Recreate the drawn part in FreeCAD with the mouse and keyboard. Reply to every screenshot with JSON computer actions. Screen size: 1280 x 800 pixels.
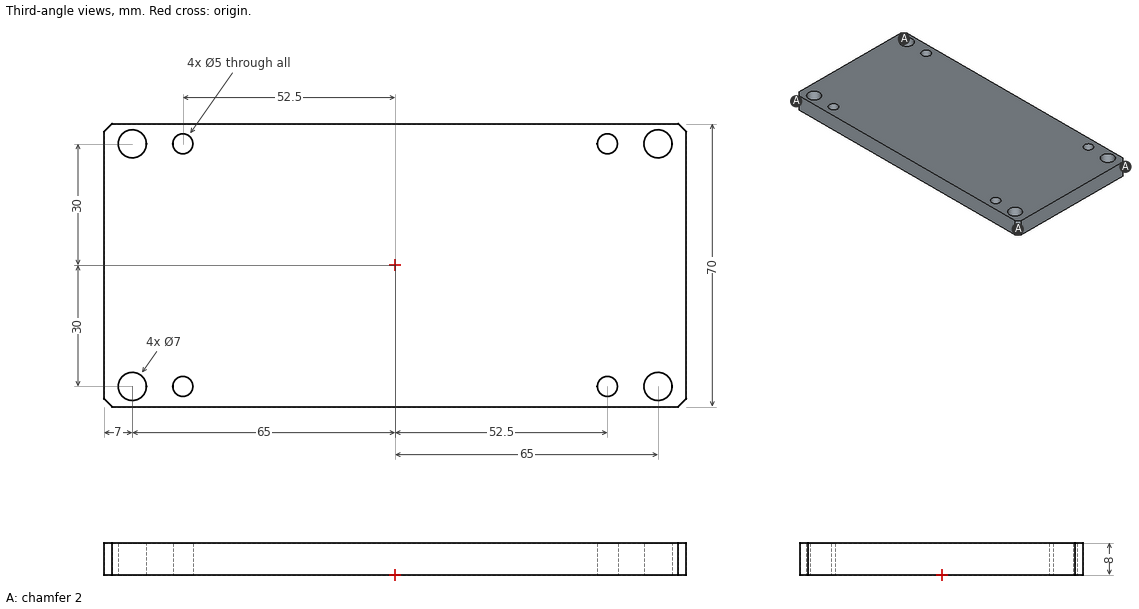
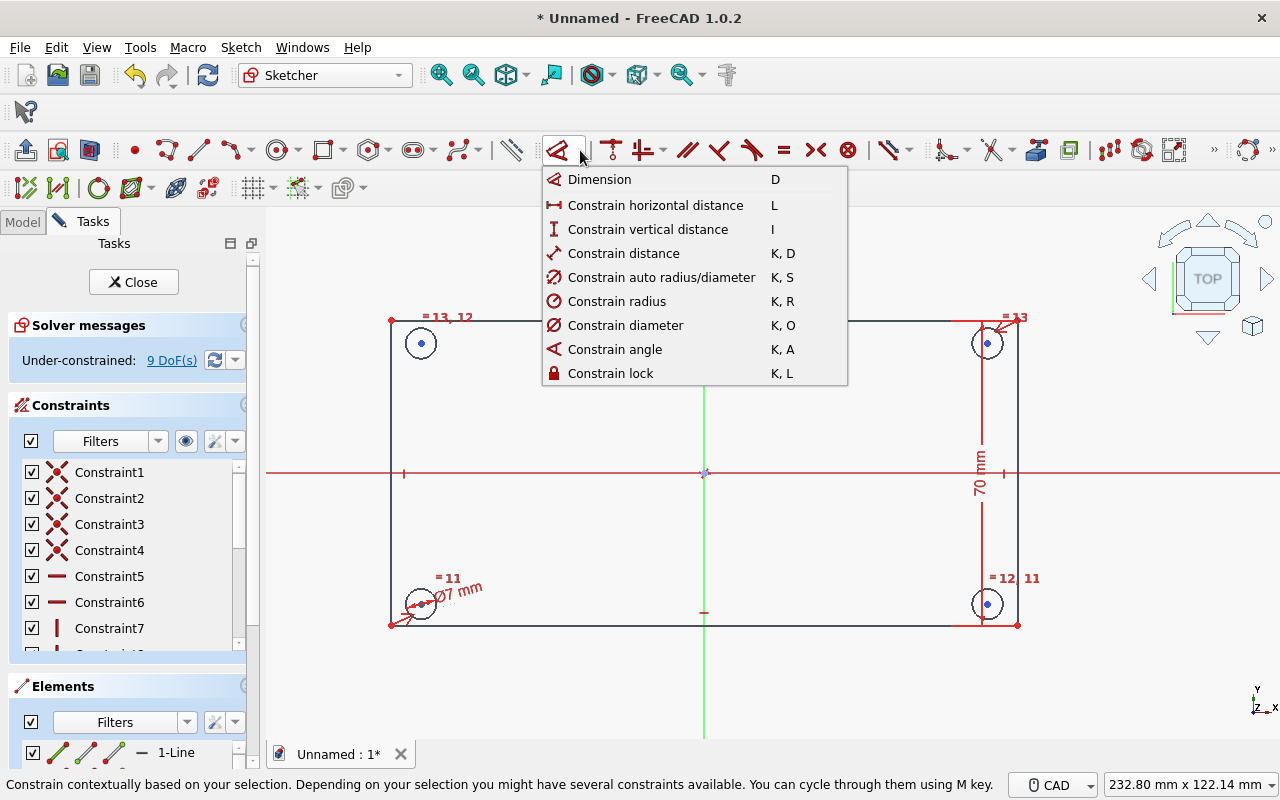
{"action": "left_click", "coordinate": [695, 205]}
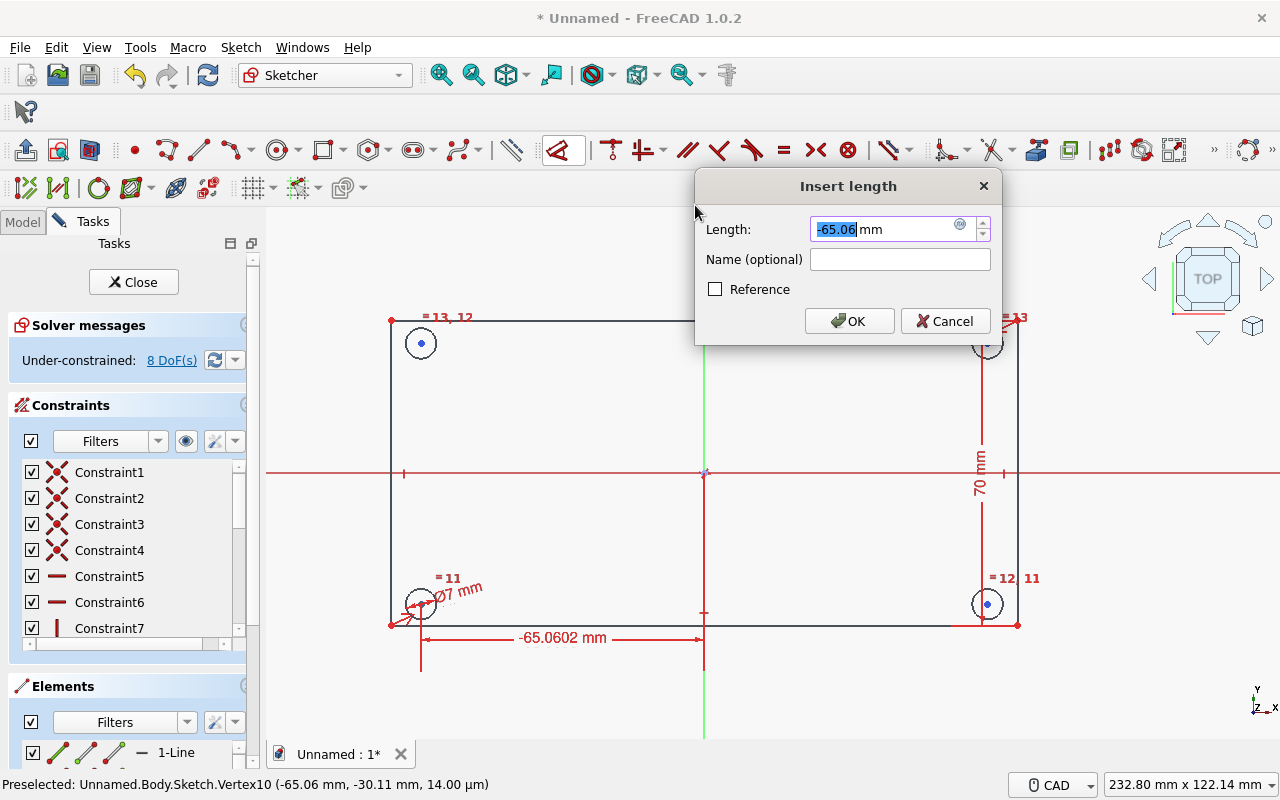
{"action": "type", "text": "-65"}
{"action": "key", "text": "Return"}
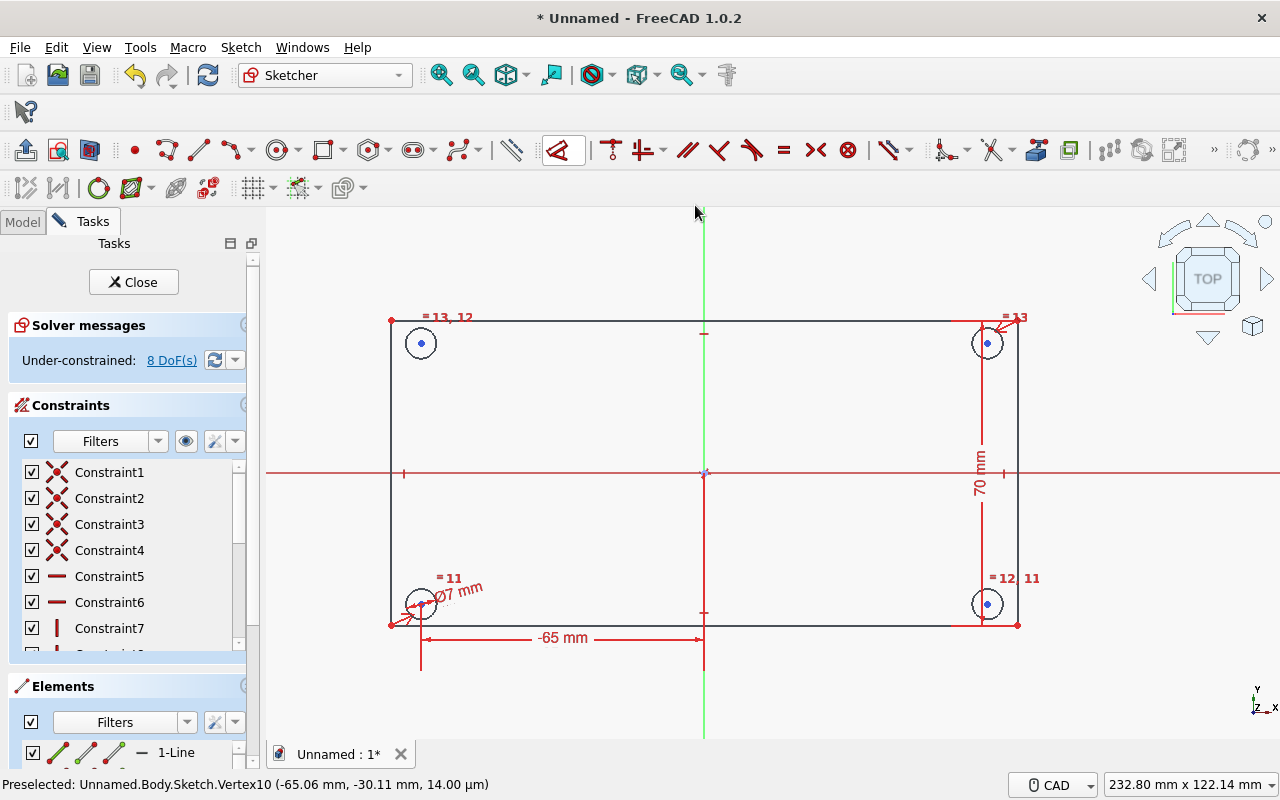
{"action": "left_click", "coordinate": [421, 604]}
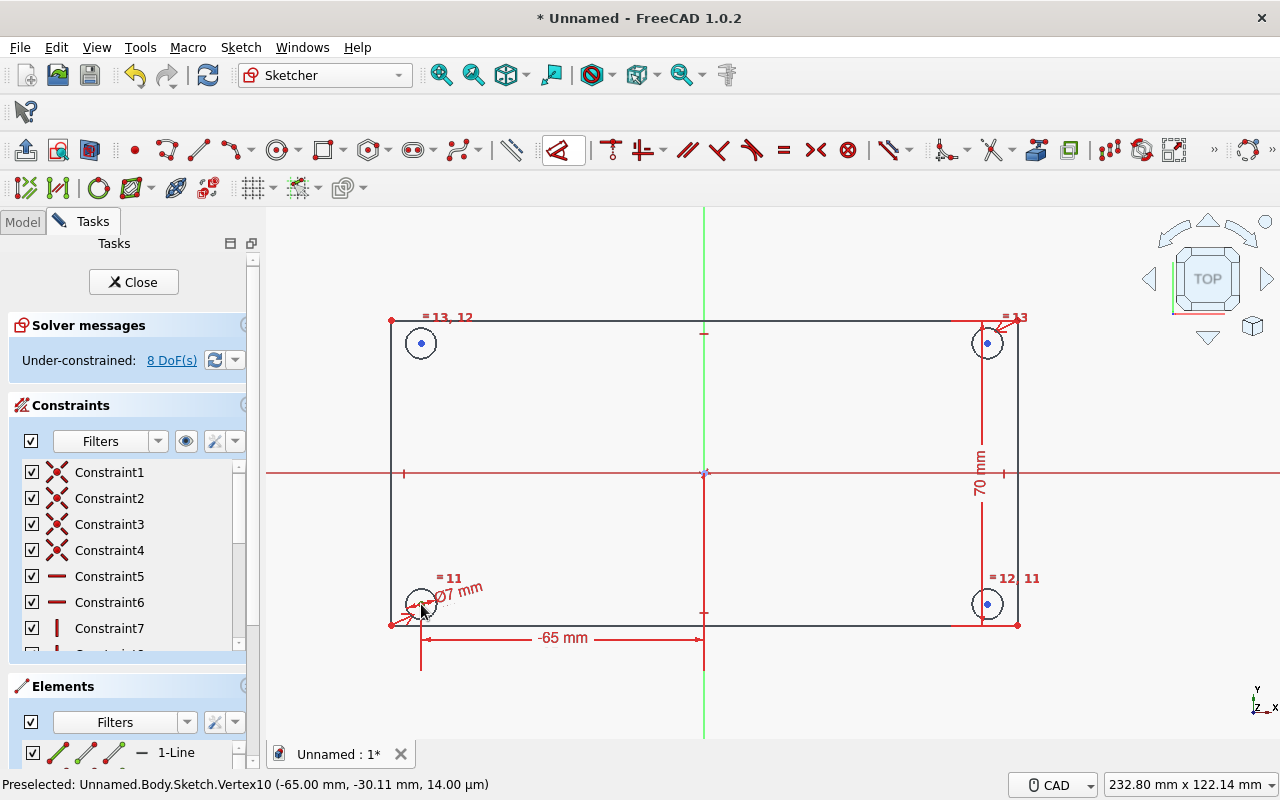
{"action": "key", "text": "i"}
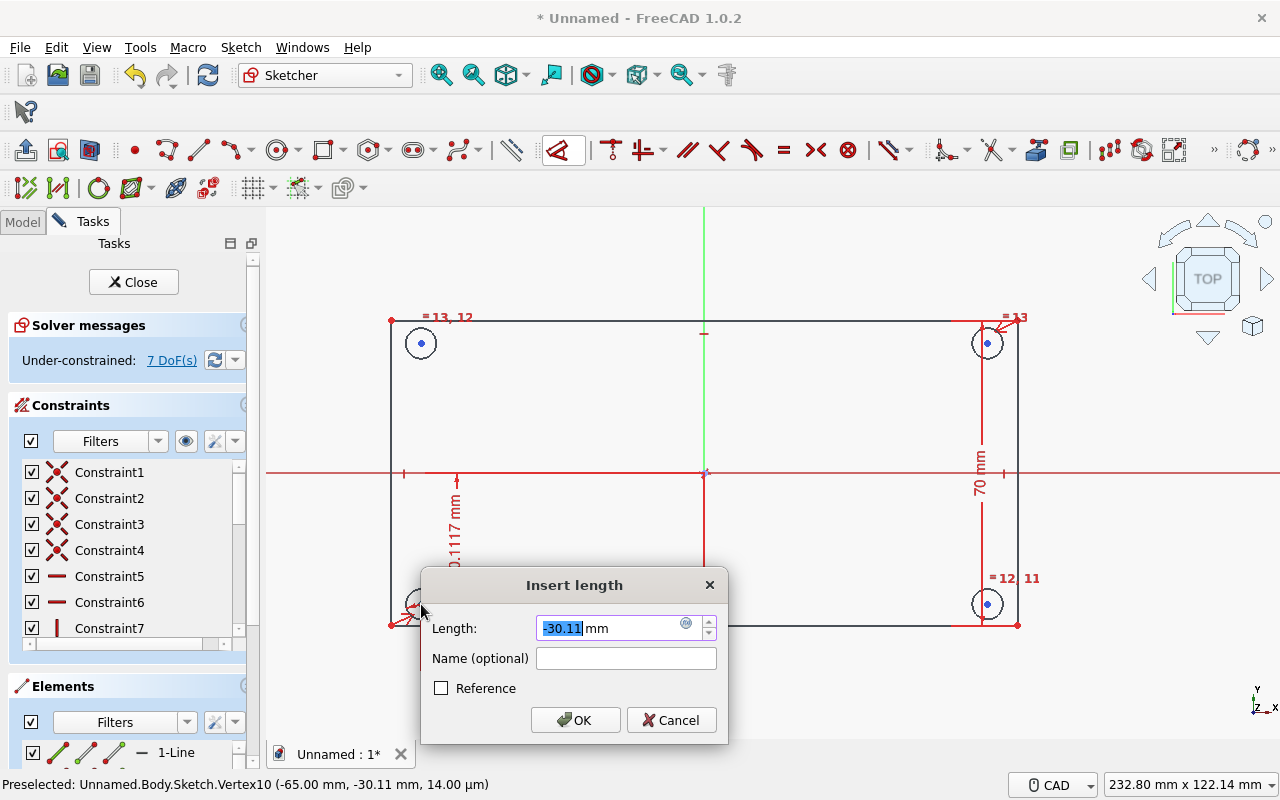
{"action": "type", "text": "-30"}
{"action": "key", "text": "Return"}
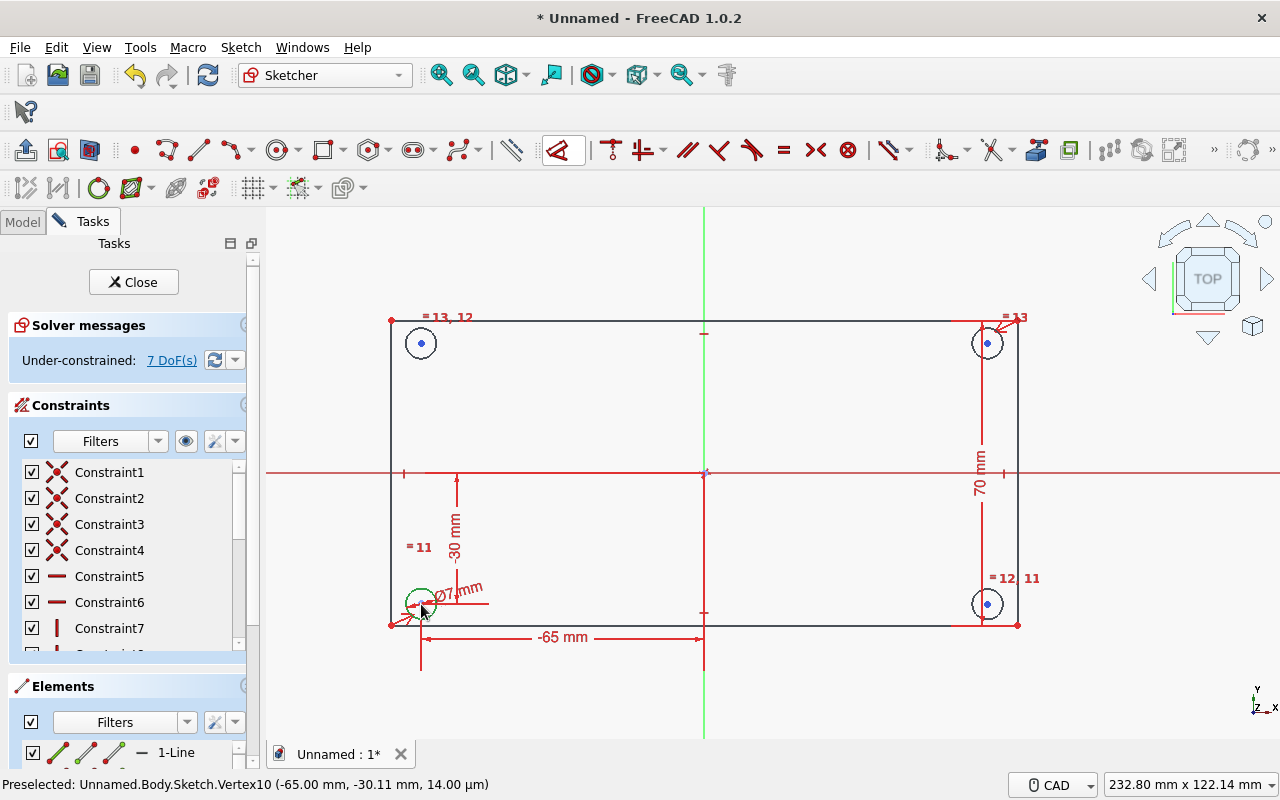
{"action": "left_click", "coordinate": [988, 604]}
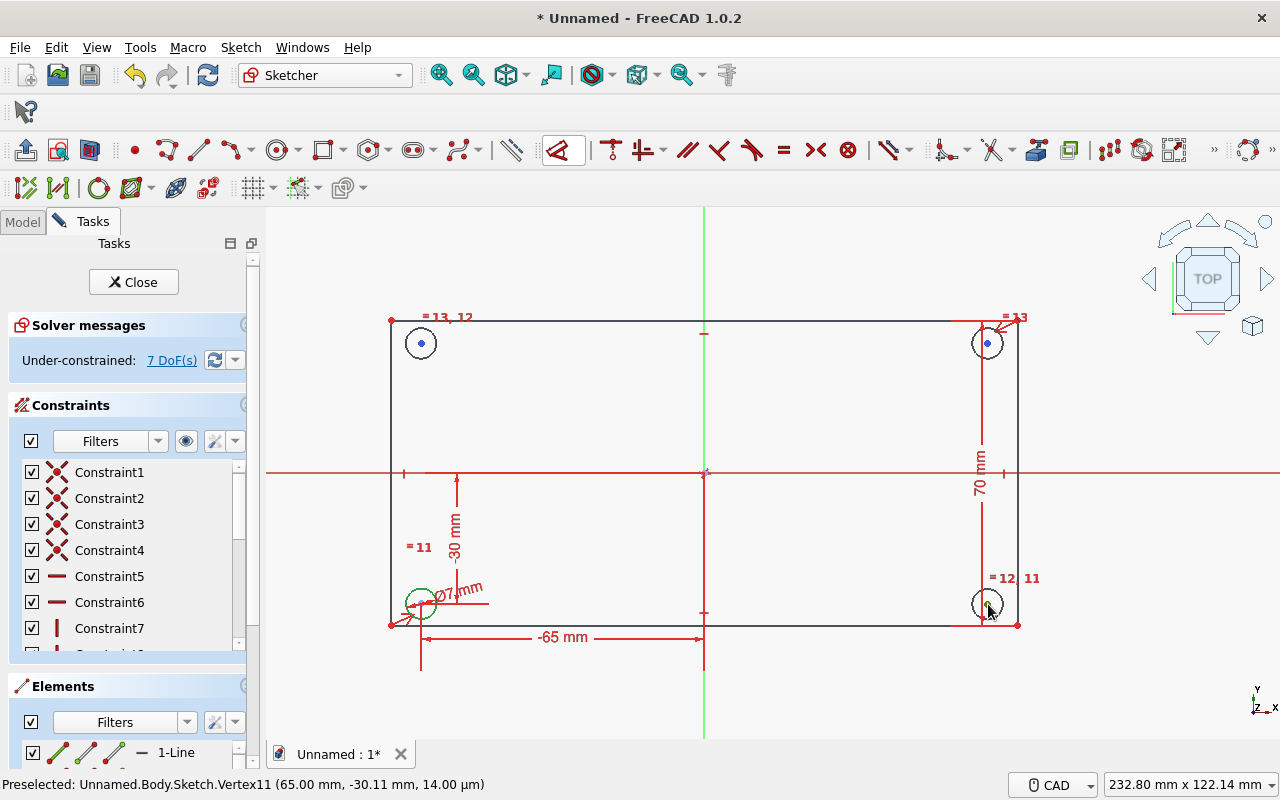
{"action": "left_click", "coordinate": [580, 150]}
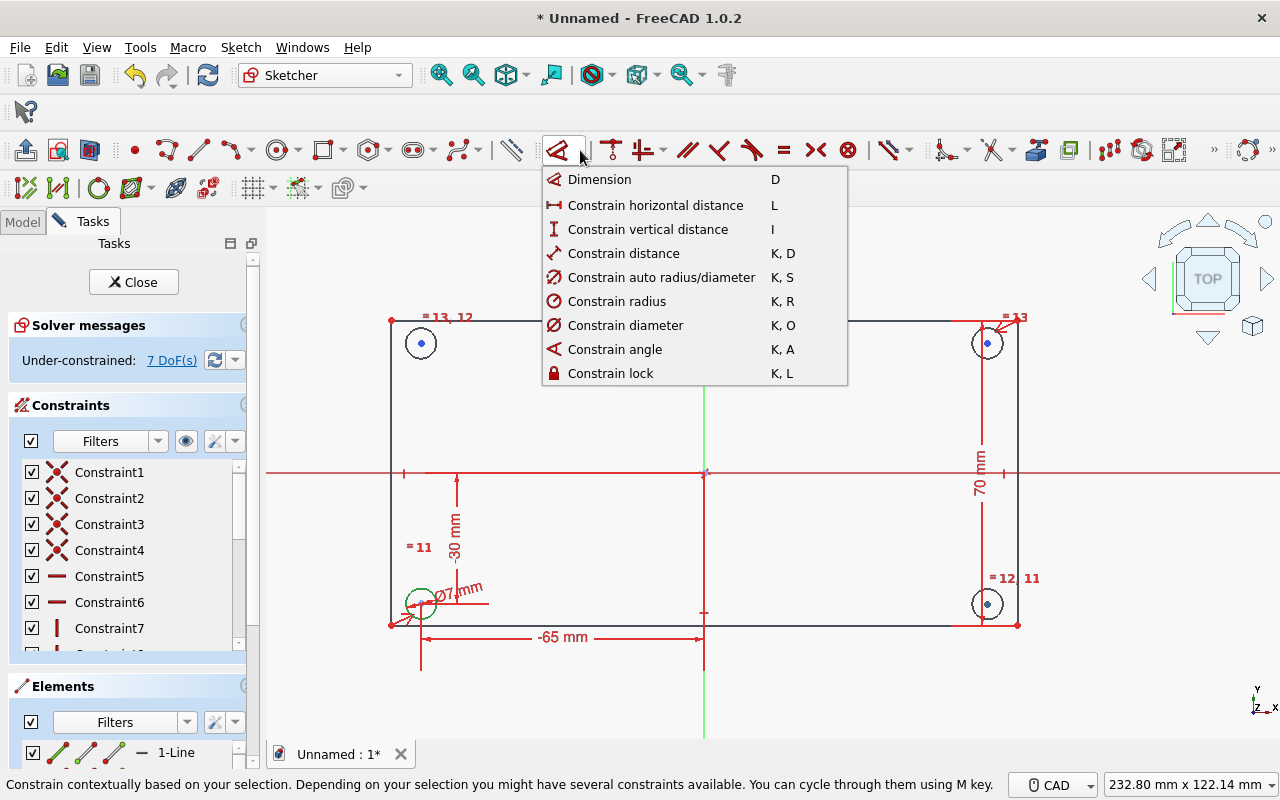
{"action": "left_click", "coordinate": [695, 205]}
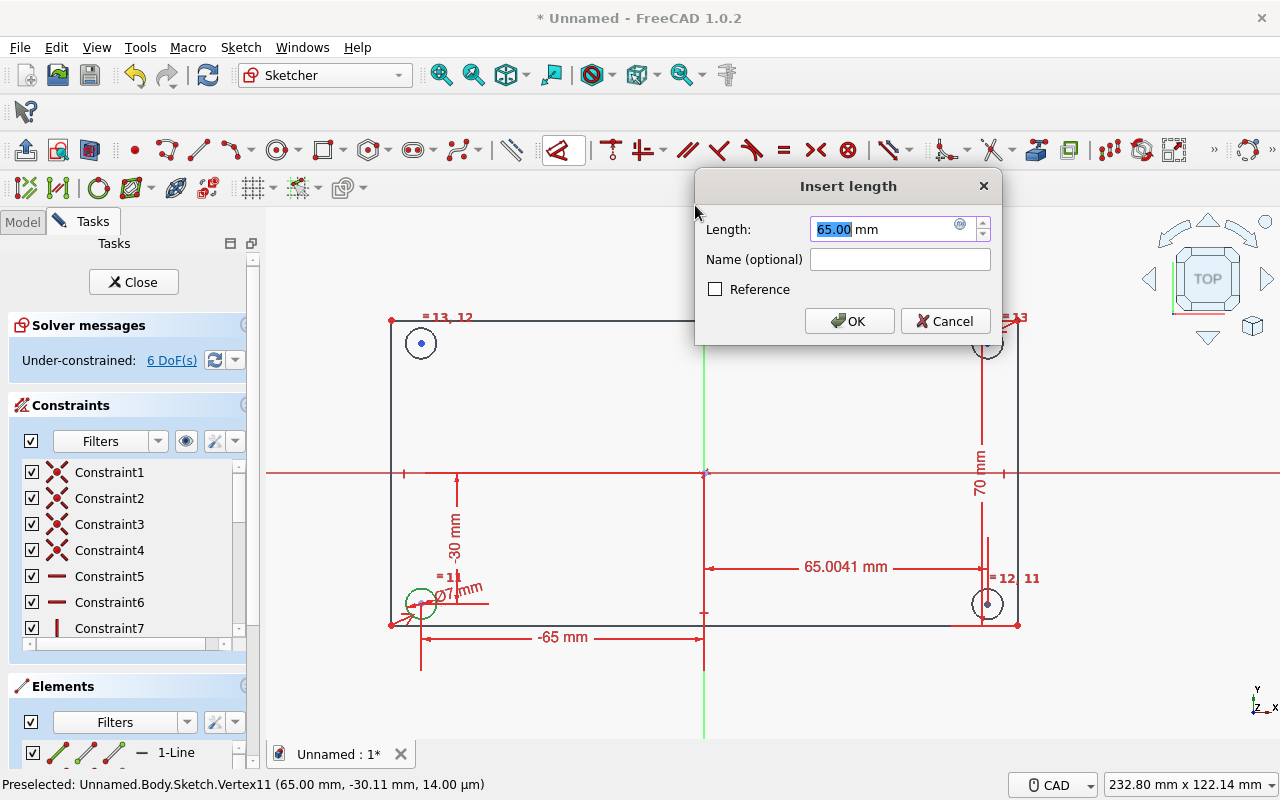
{"action": "type", "text": "65"}
{"action": "key", "text": "Return"}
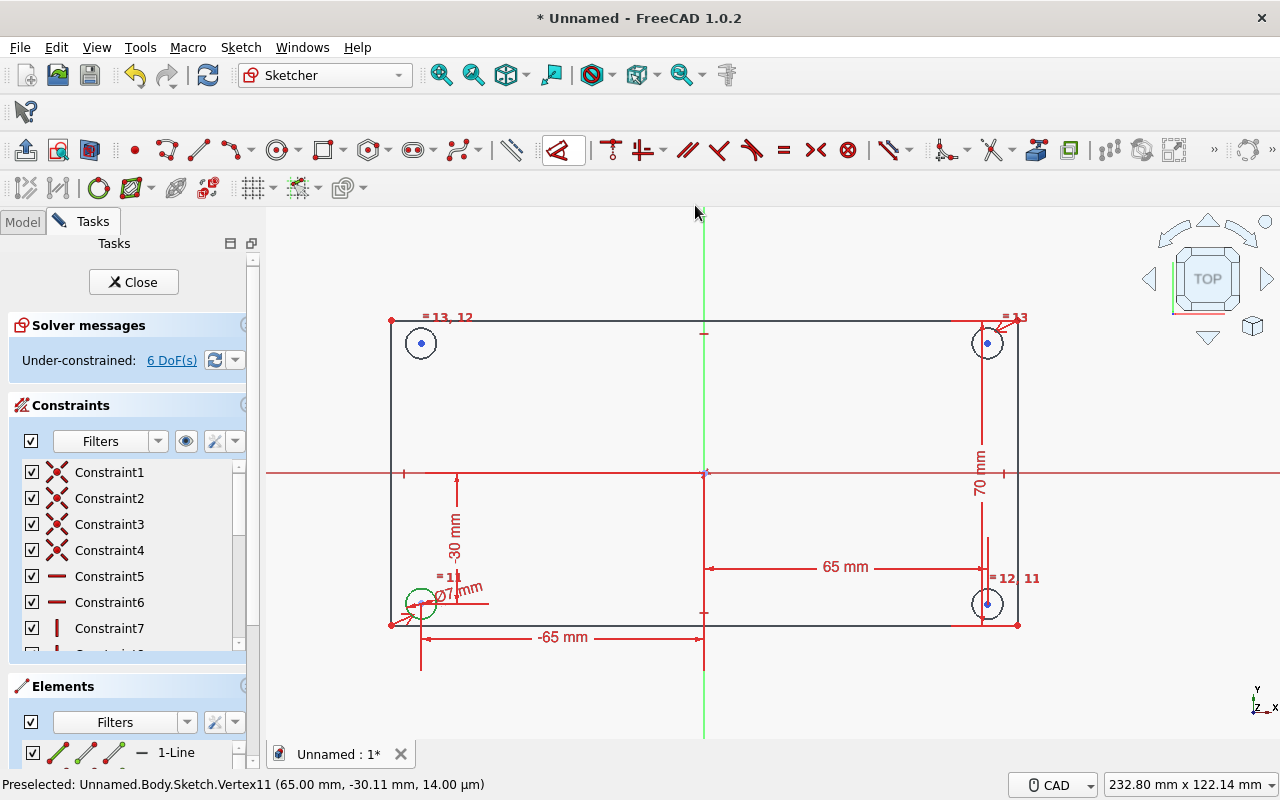
{"action": "left_click", "coordinate": [988, 604]}